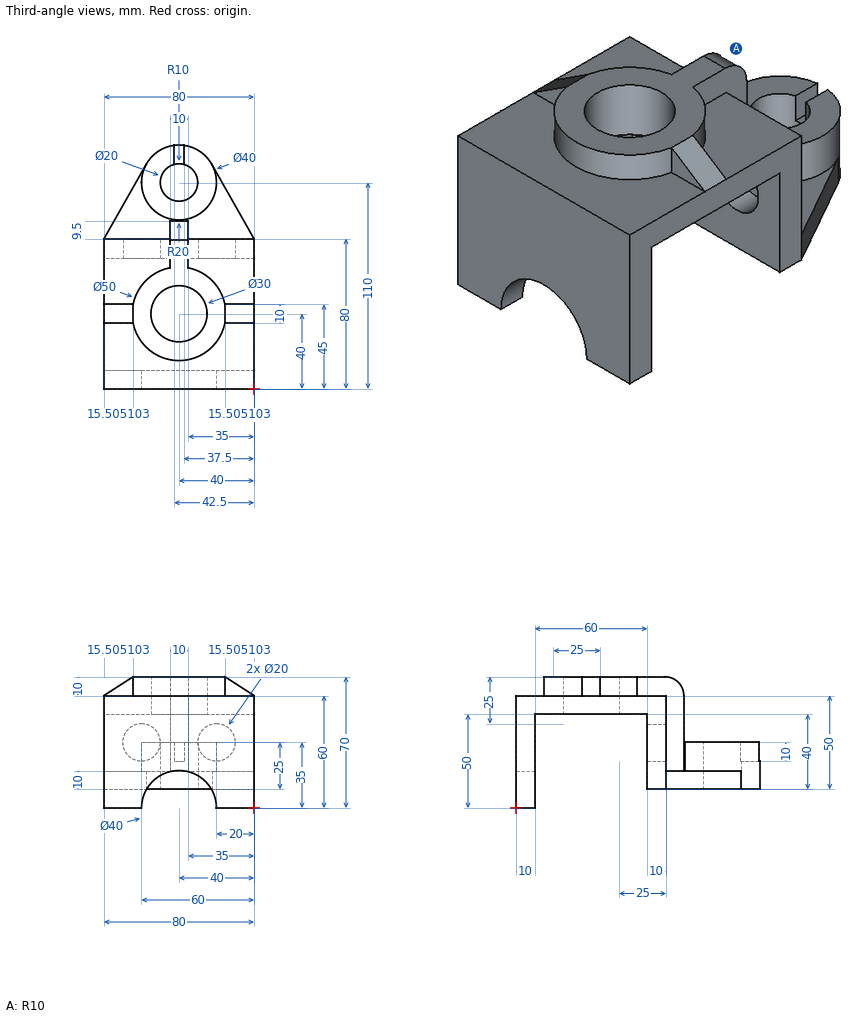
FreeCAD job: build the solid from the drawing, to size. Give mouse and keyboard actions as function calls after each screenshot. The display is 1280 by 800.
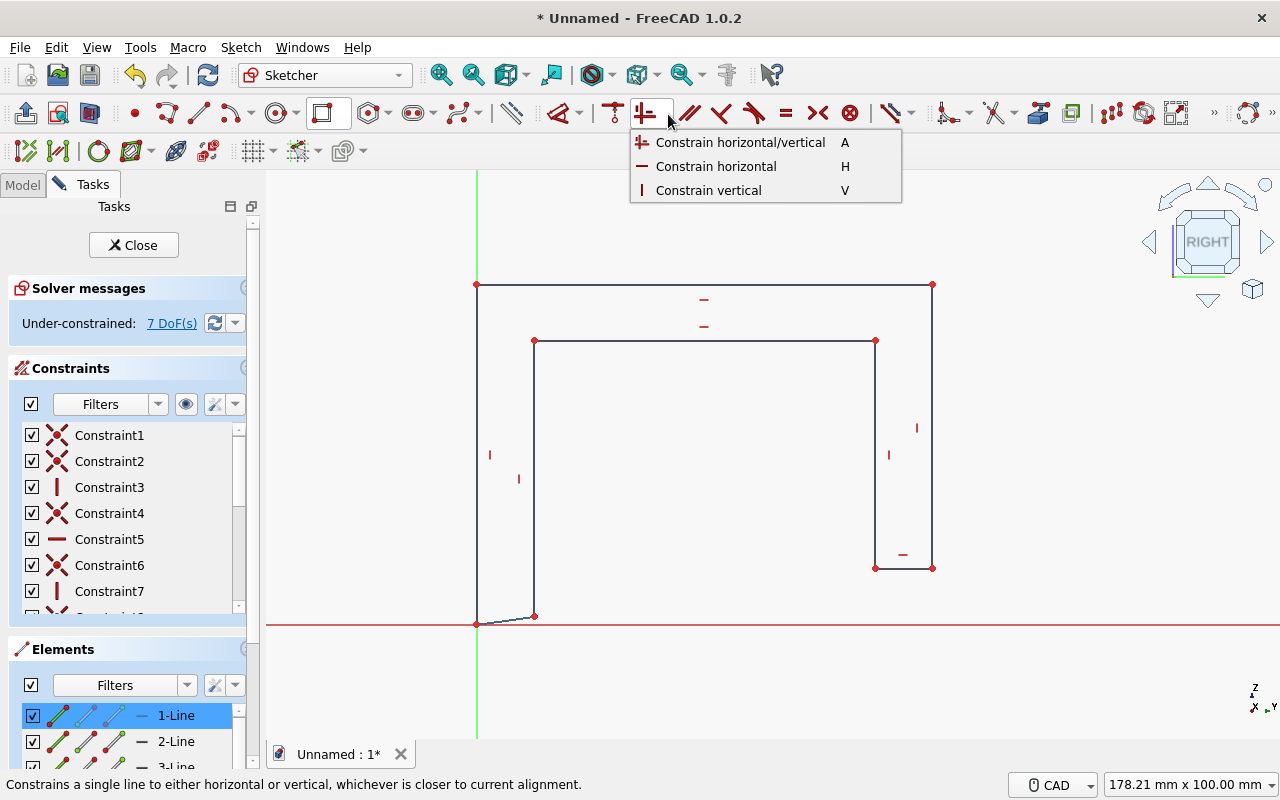
click(766, 166)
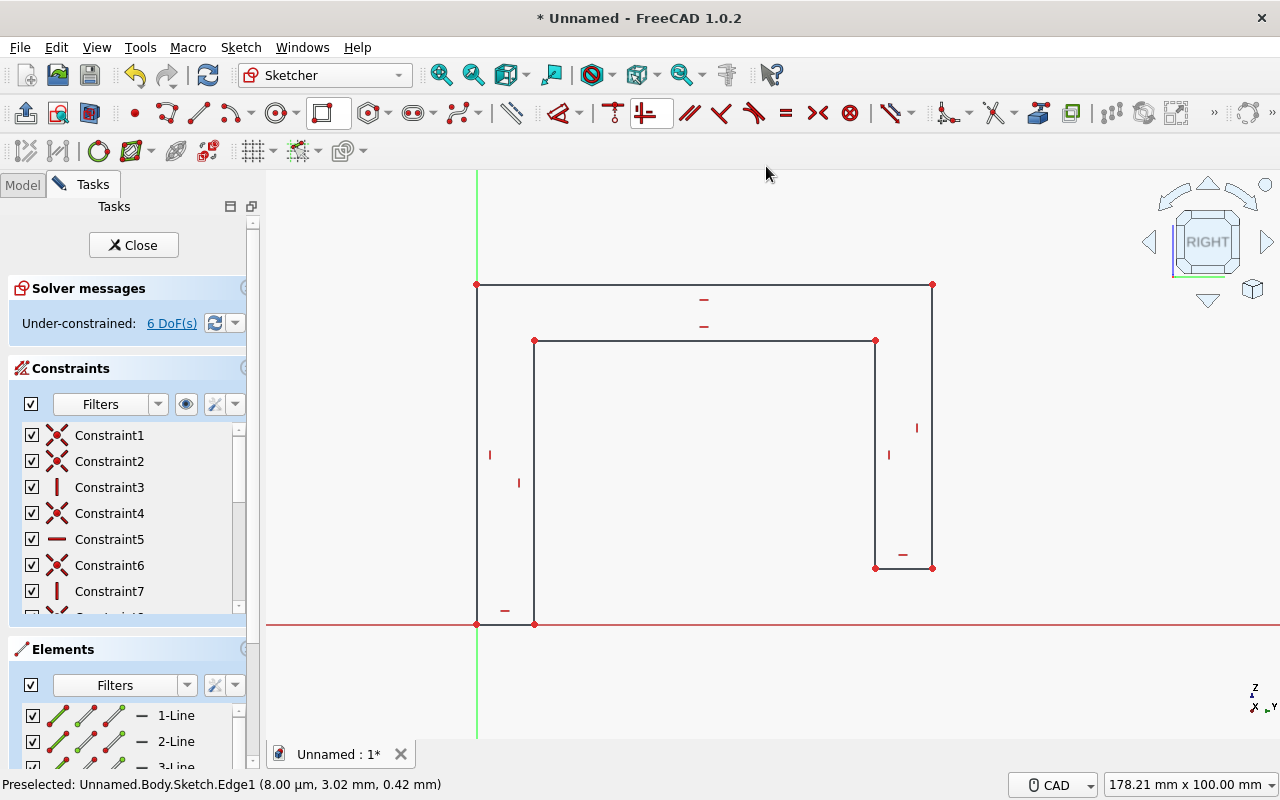
click(558, 114)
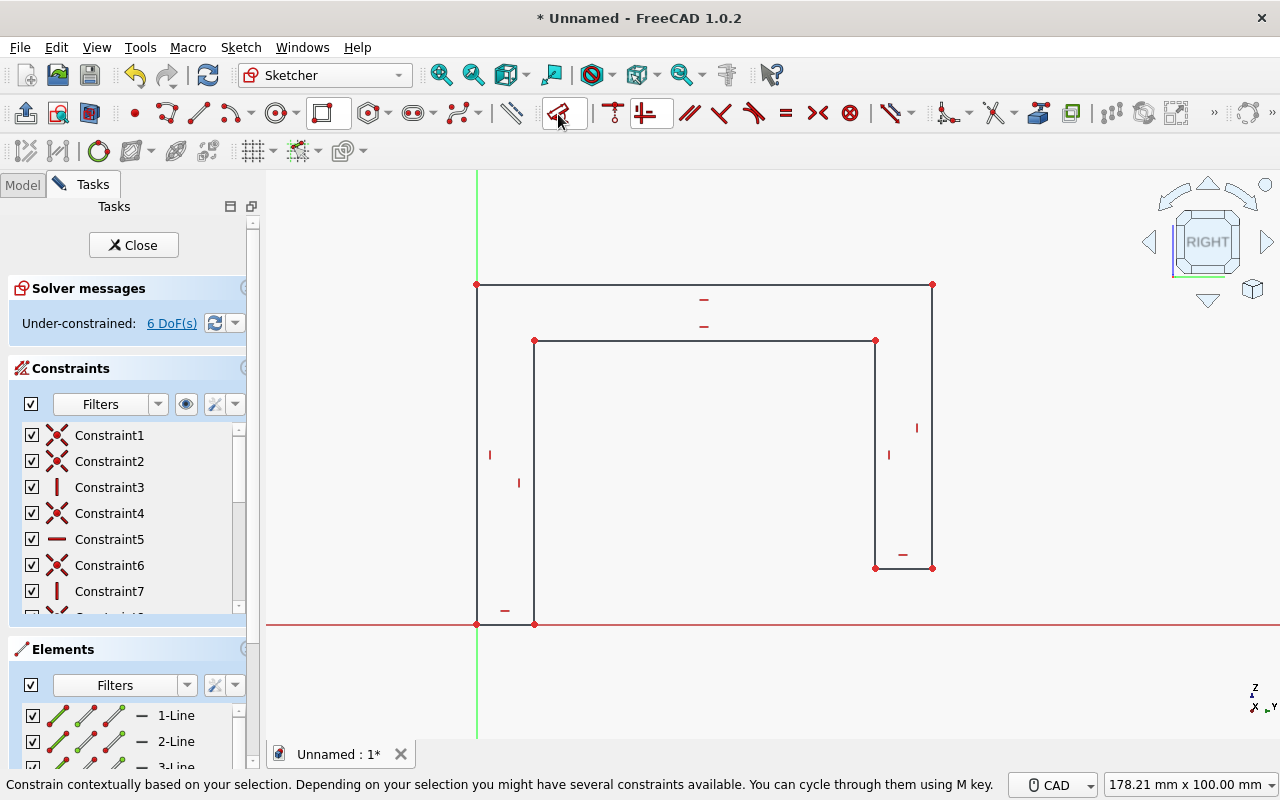
click(494, 625)
click(505, 659)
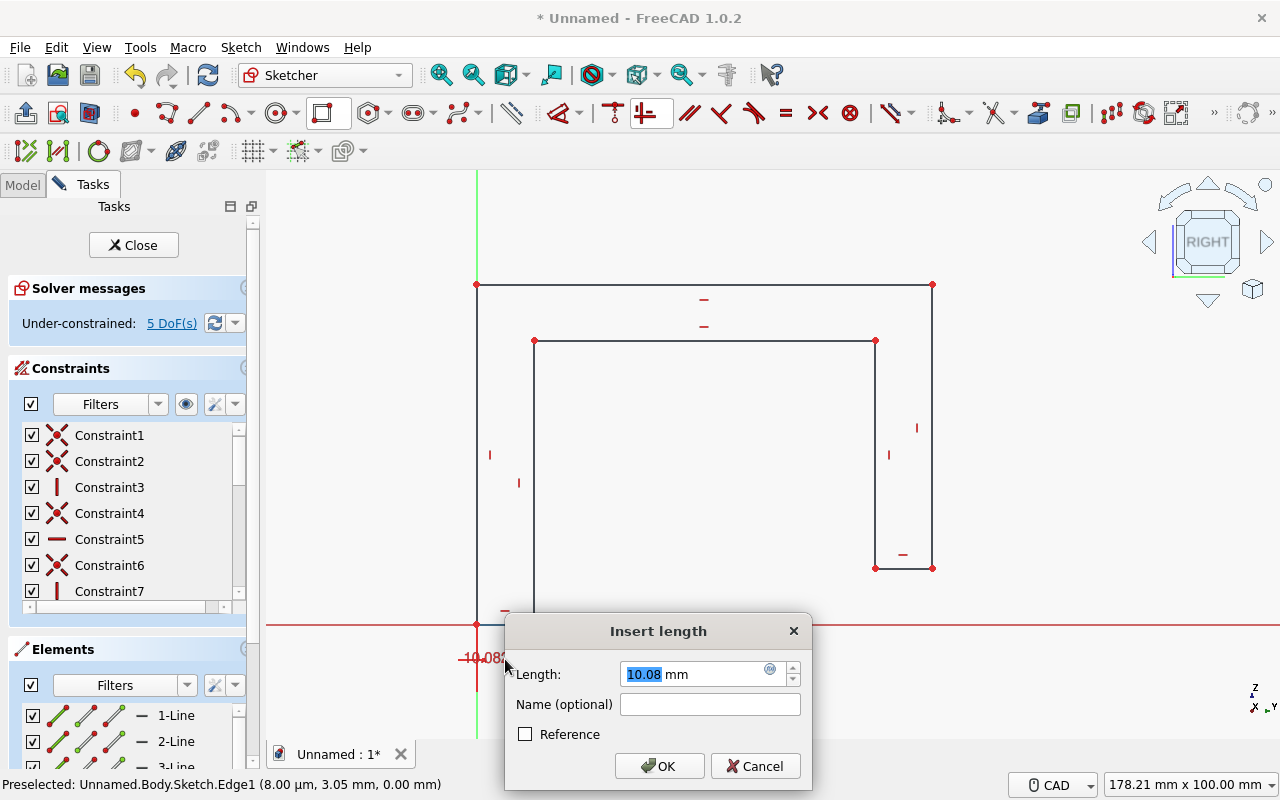
text(10)
key(Return)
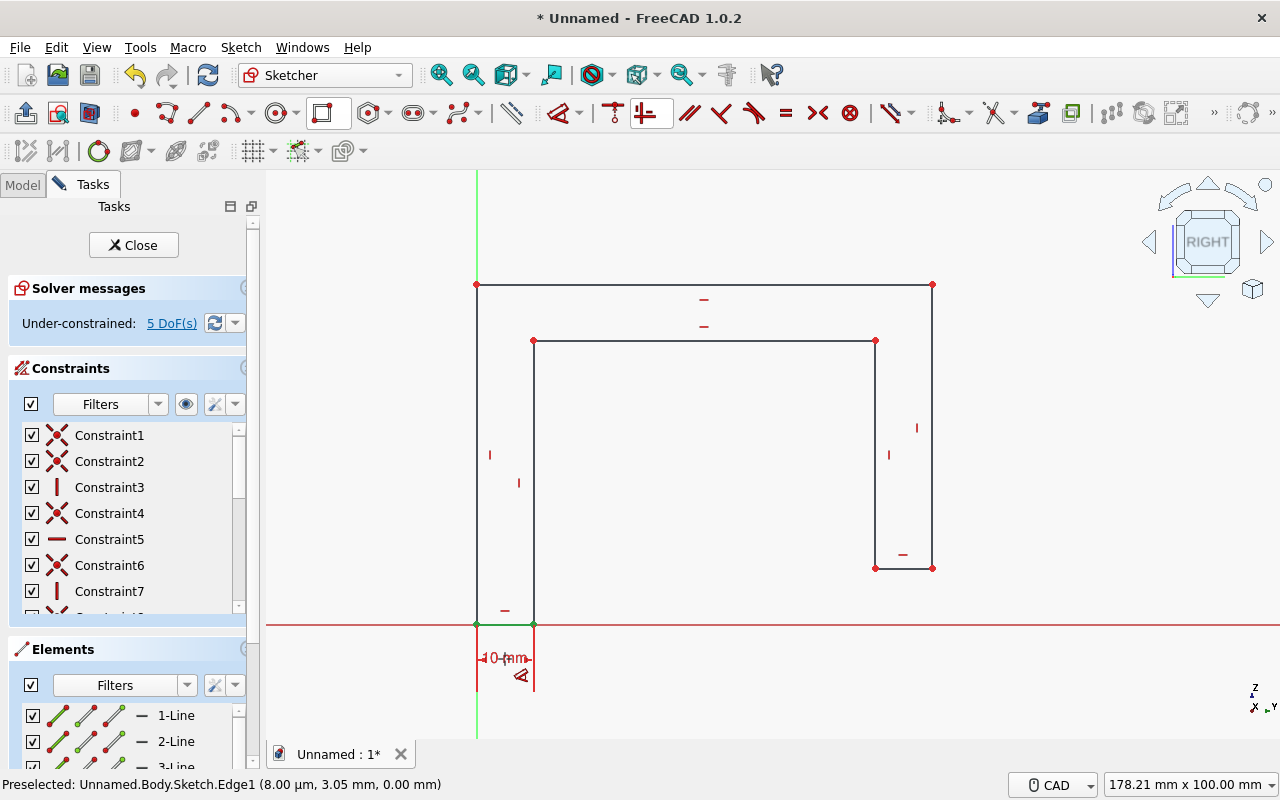
click(534, 540)
click(500, 483)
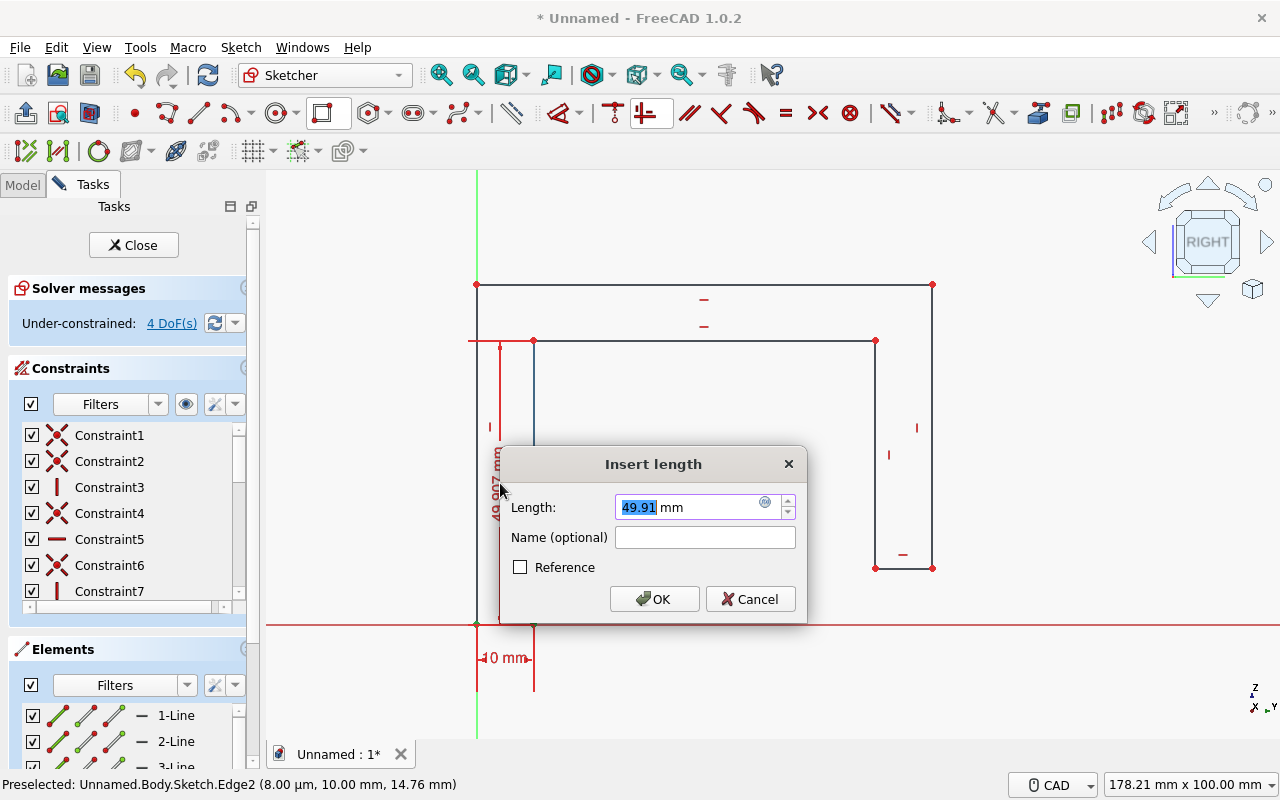
text(50)
key(Return)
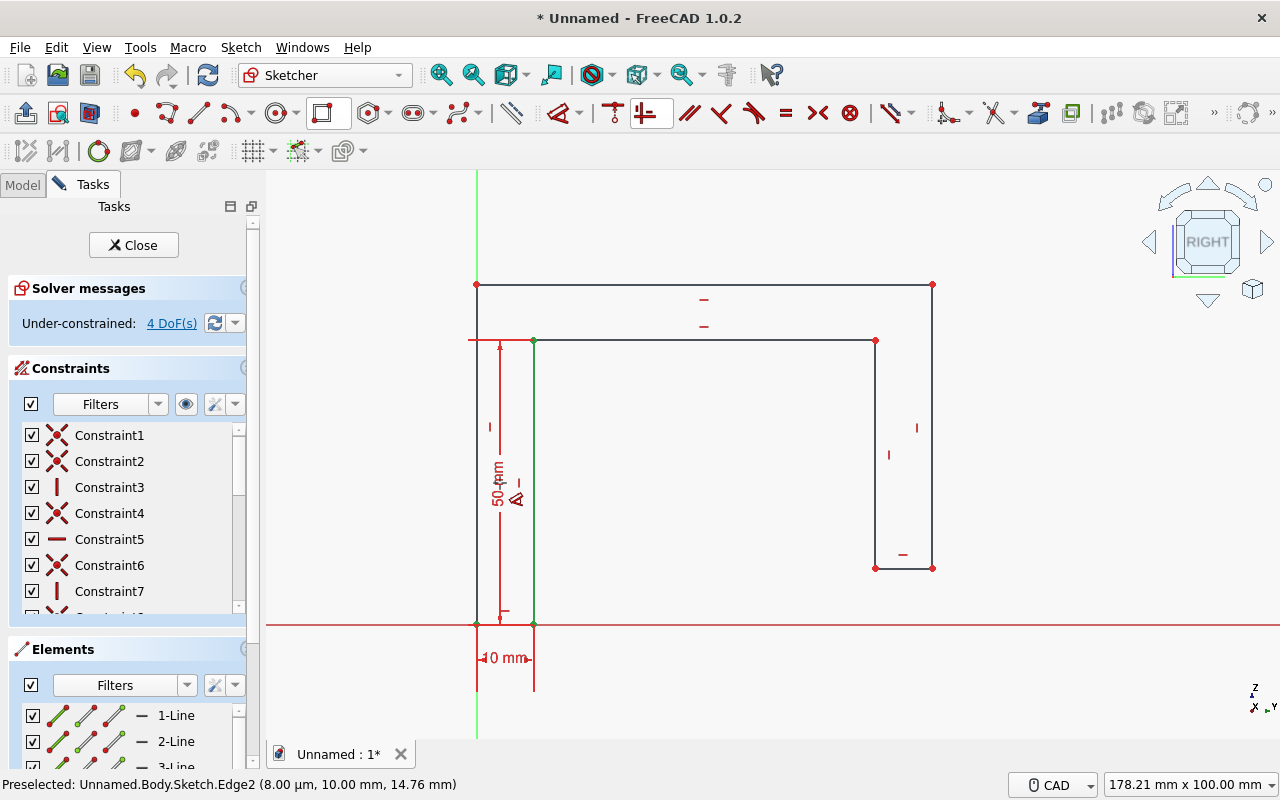
click(636, 340)
click(704, 306)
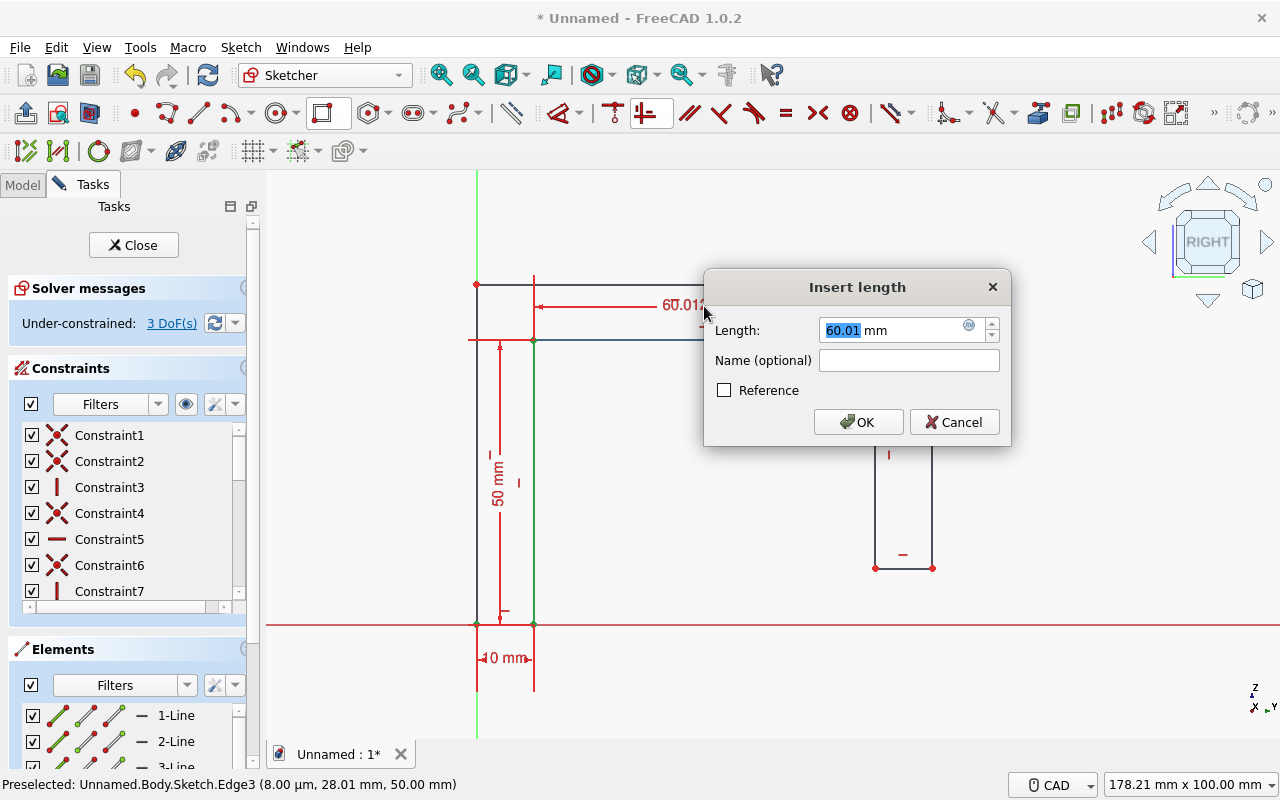
text(60)
key(Return)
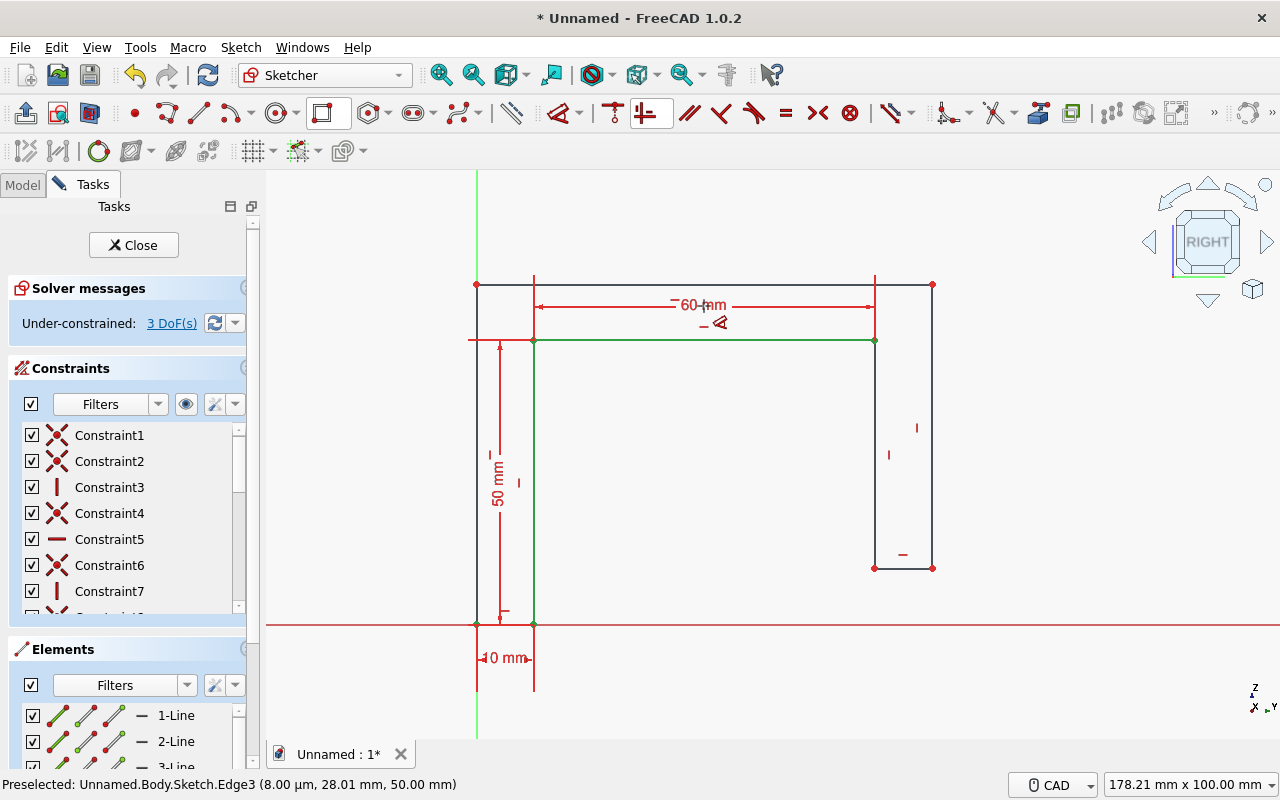
click(875, 409)
click(909, 455)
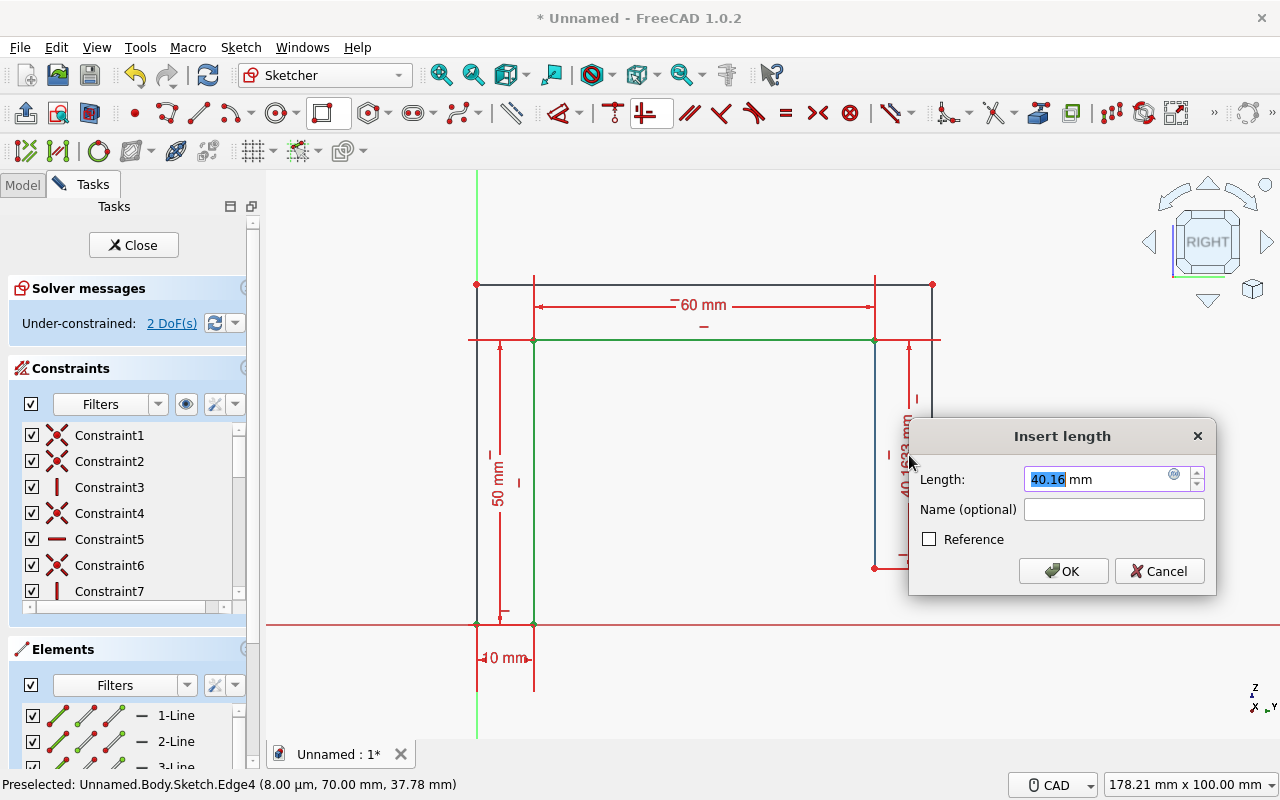
text(40)
key(Return)